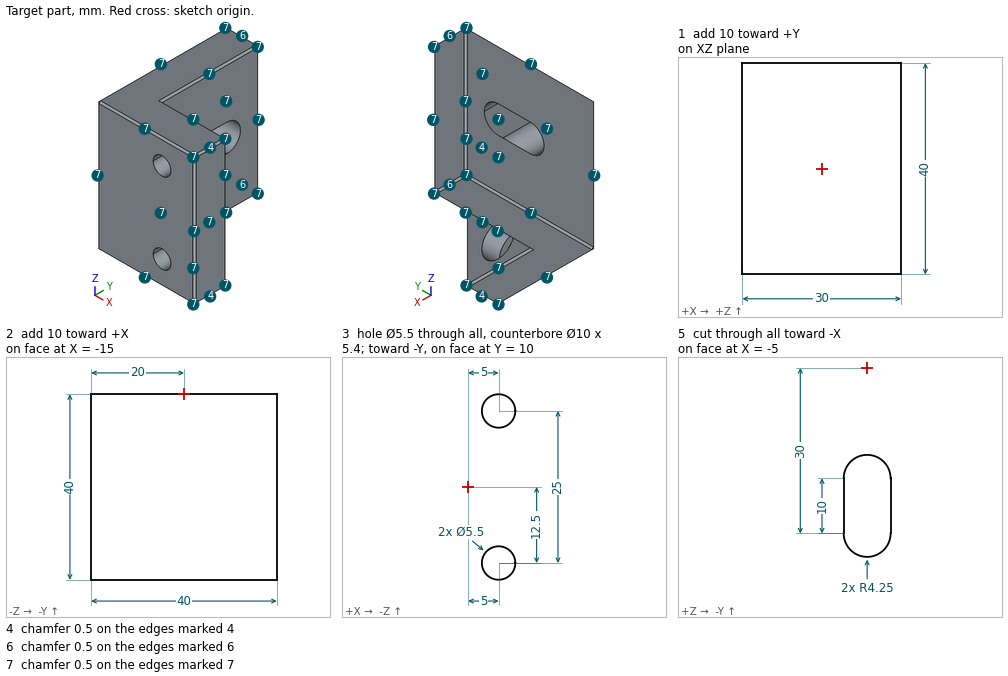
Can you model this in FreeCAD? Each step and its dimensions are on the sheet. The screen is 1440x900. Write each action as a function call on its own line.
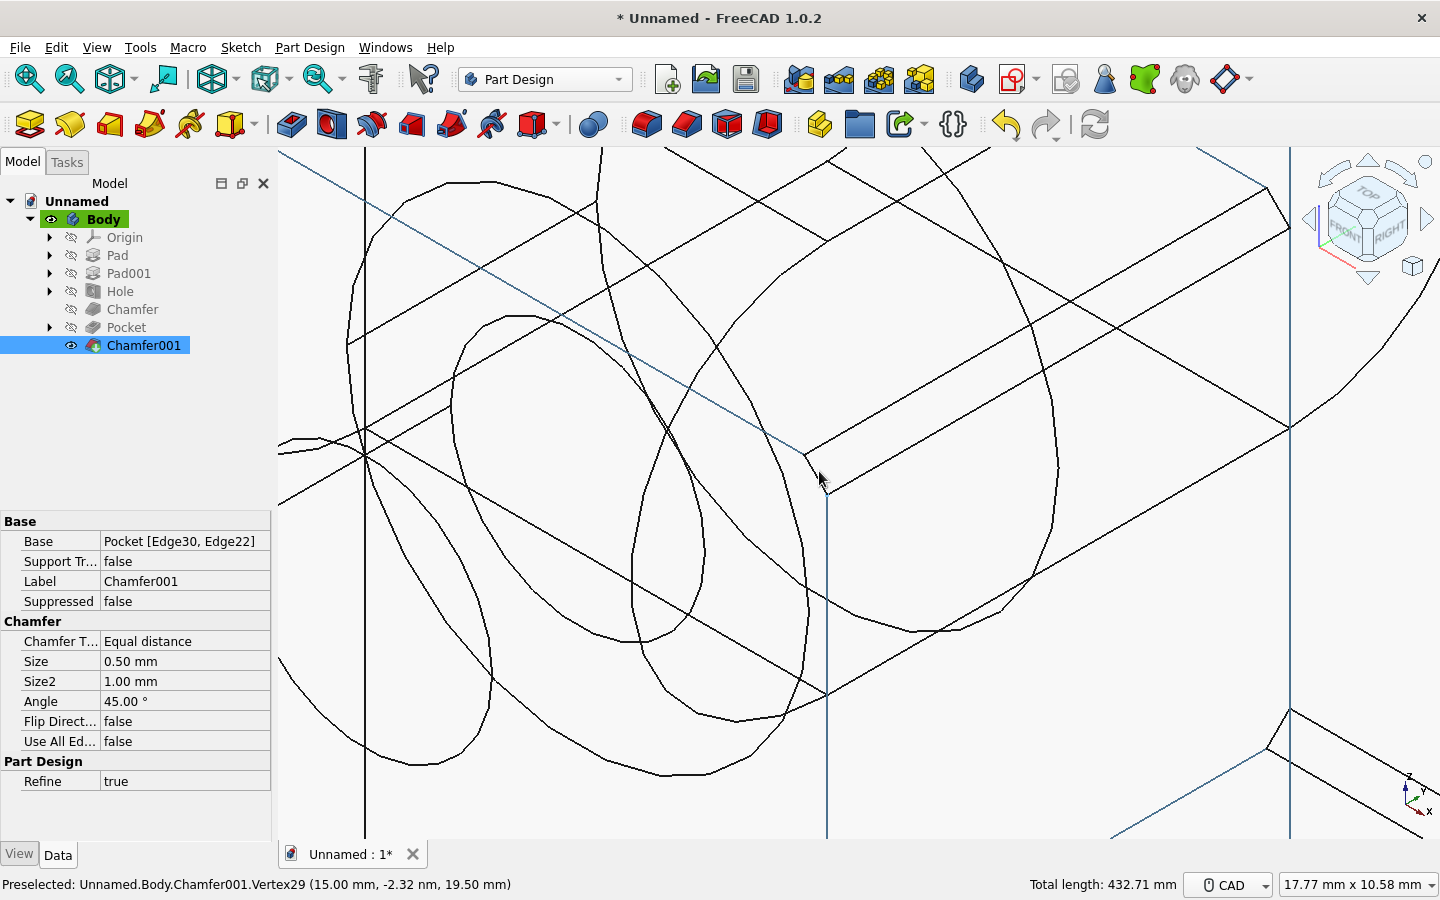
click(816, 474, ctrl)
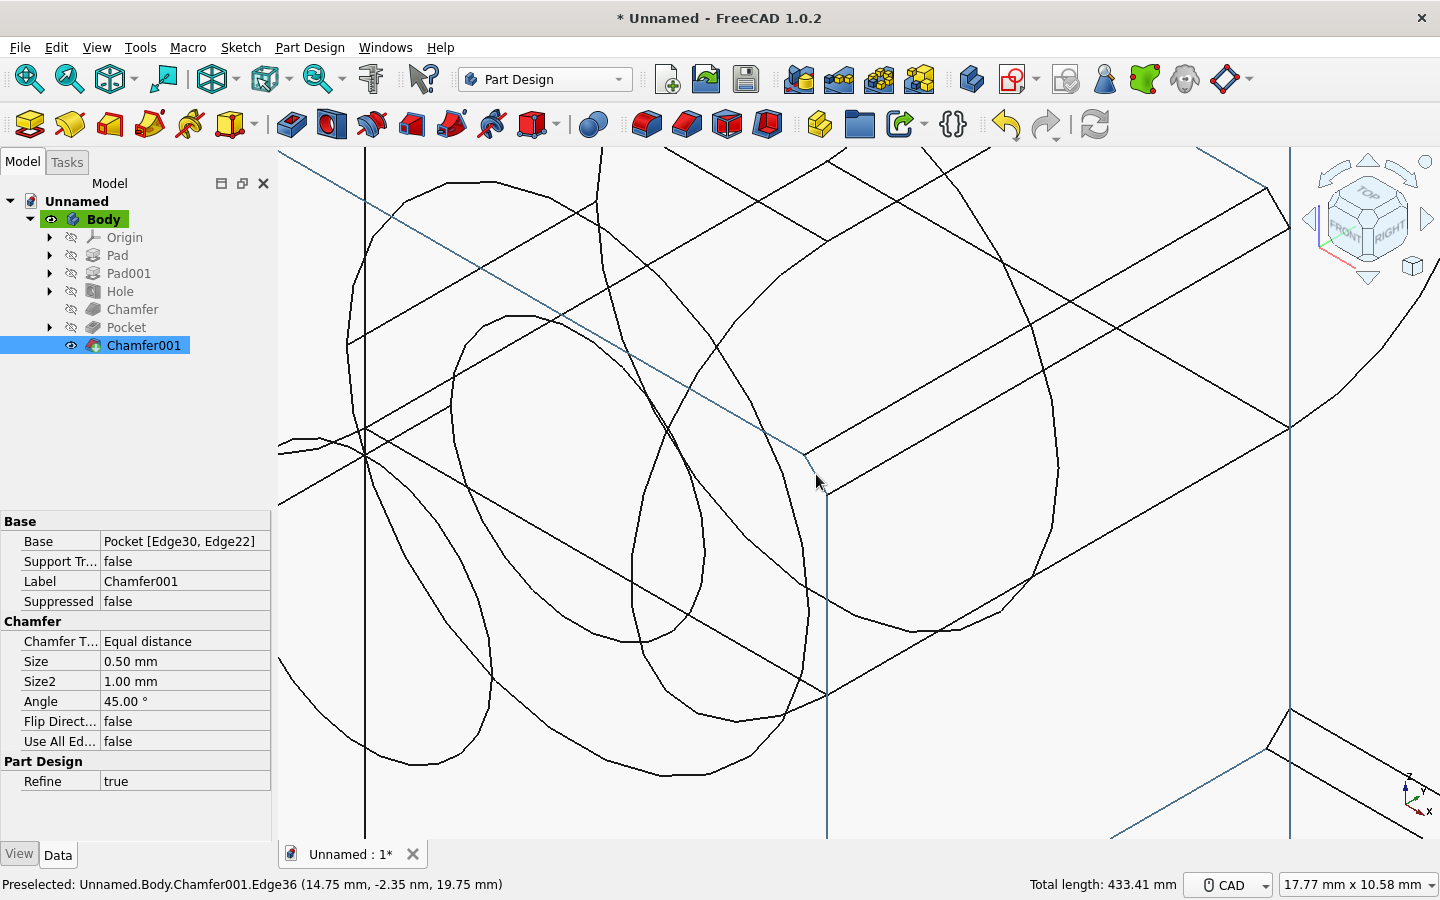
click(1274, 199, ctrl)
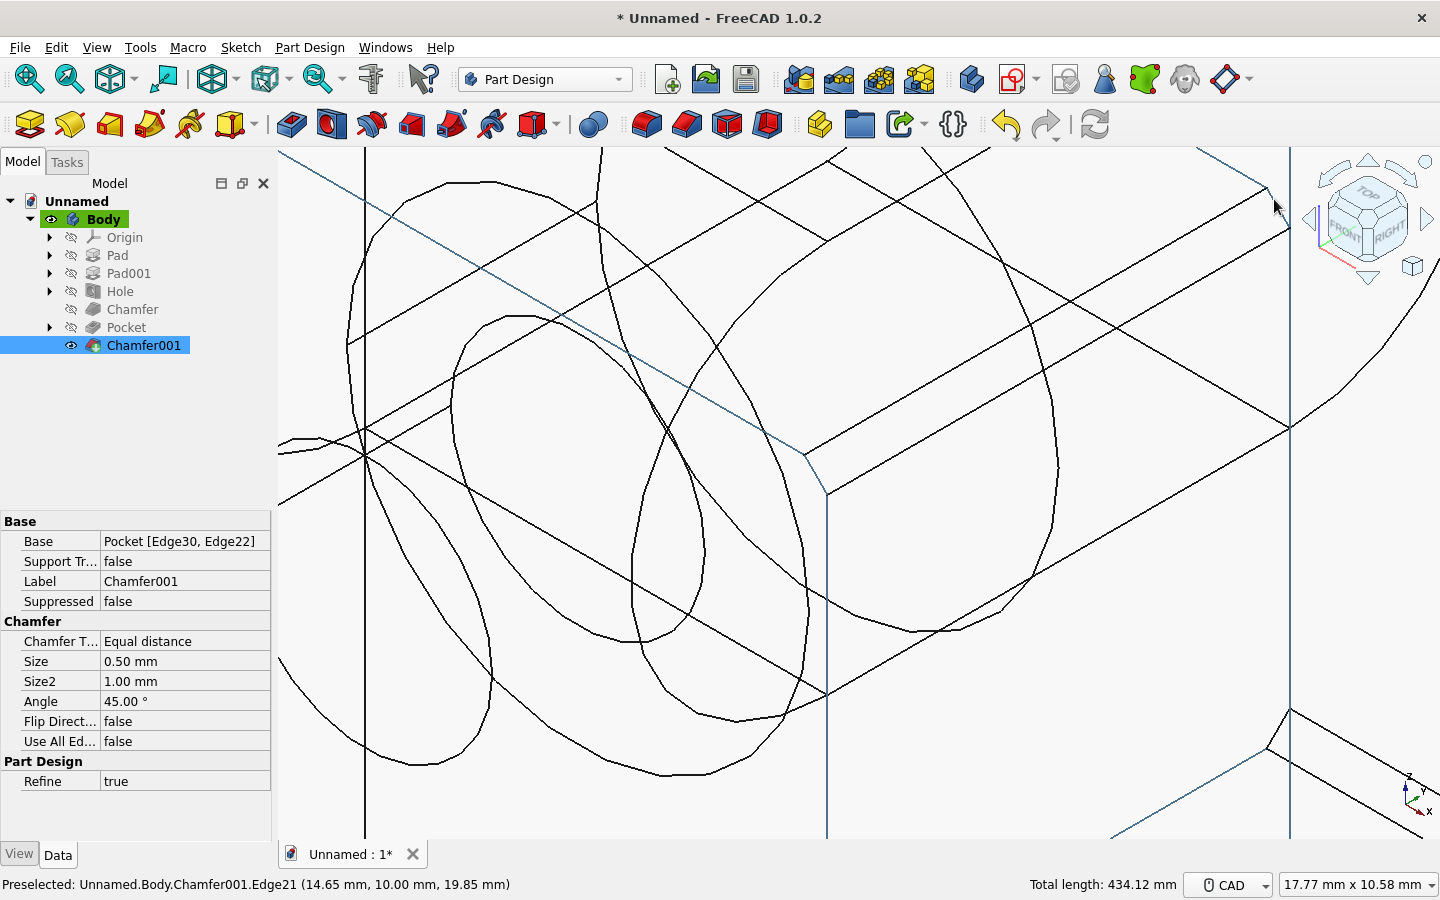
click(1278, 728, ctrl)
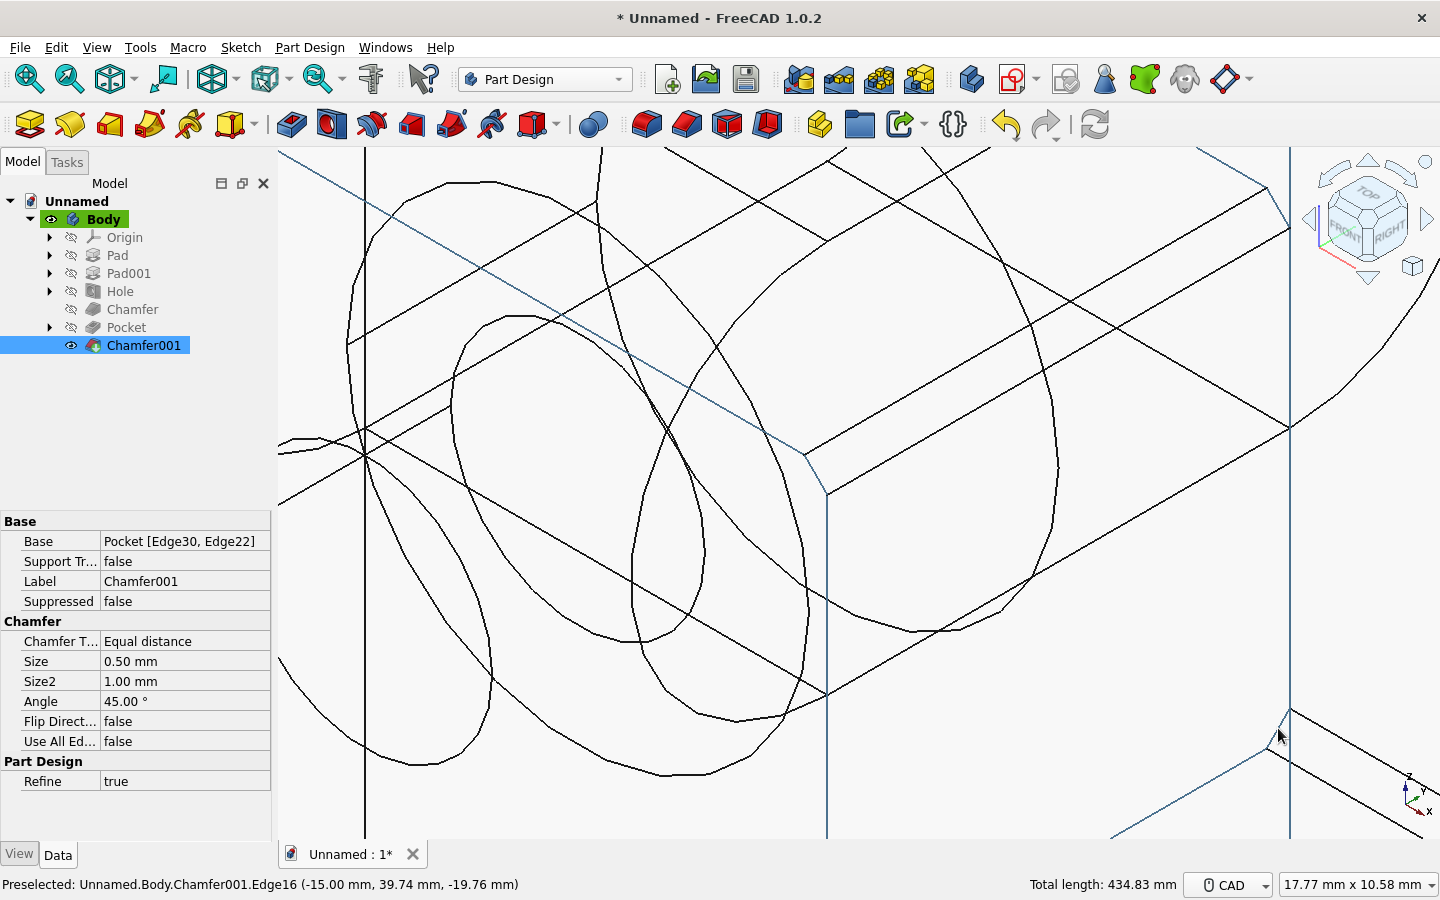
click(30, 80)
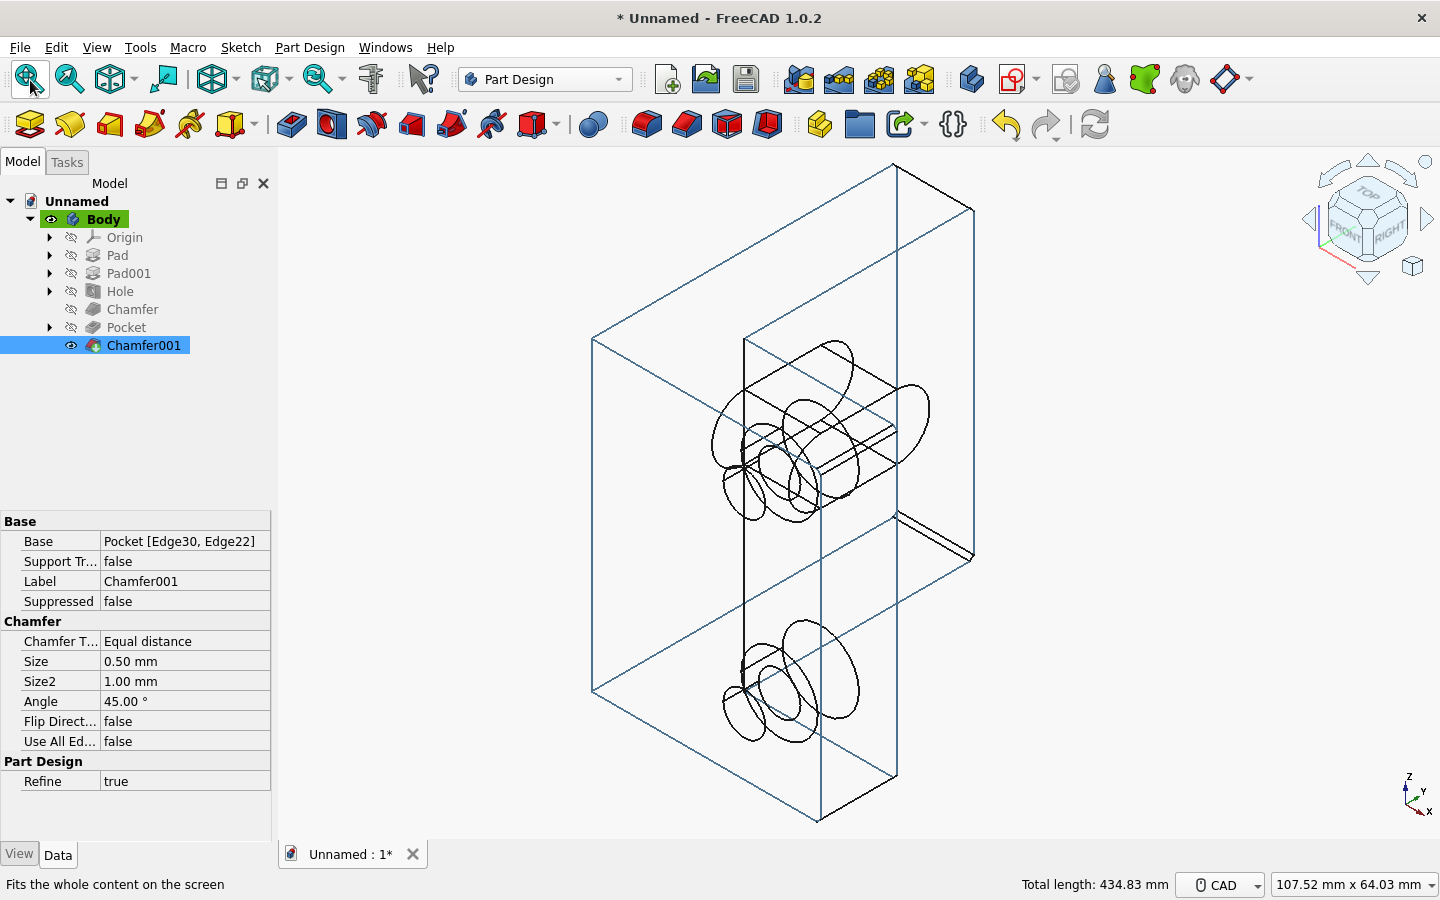
key(2)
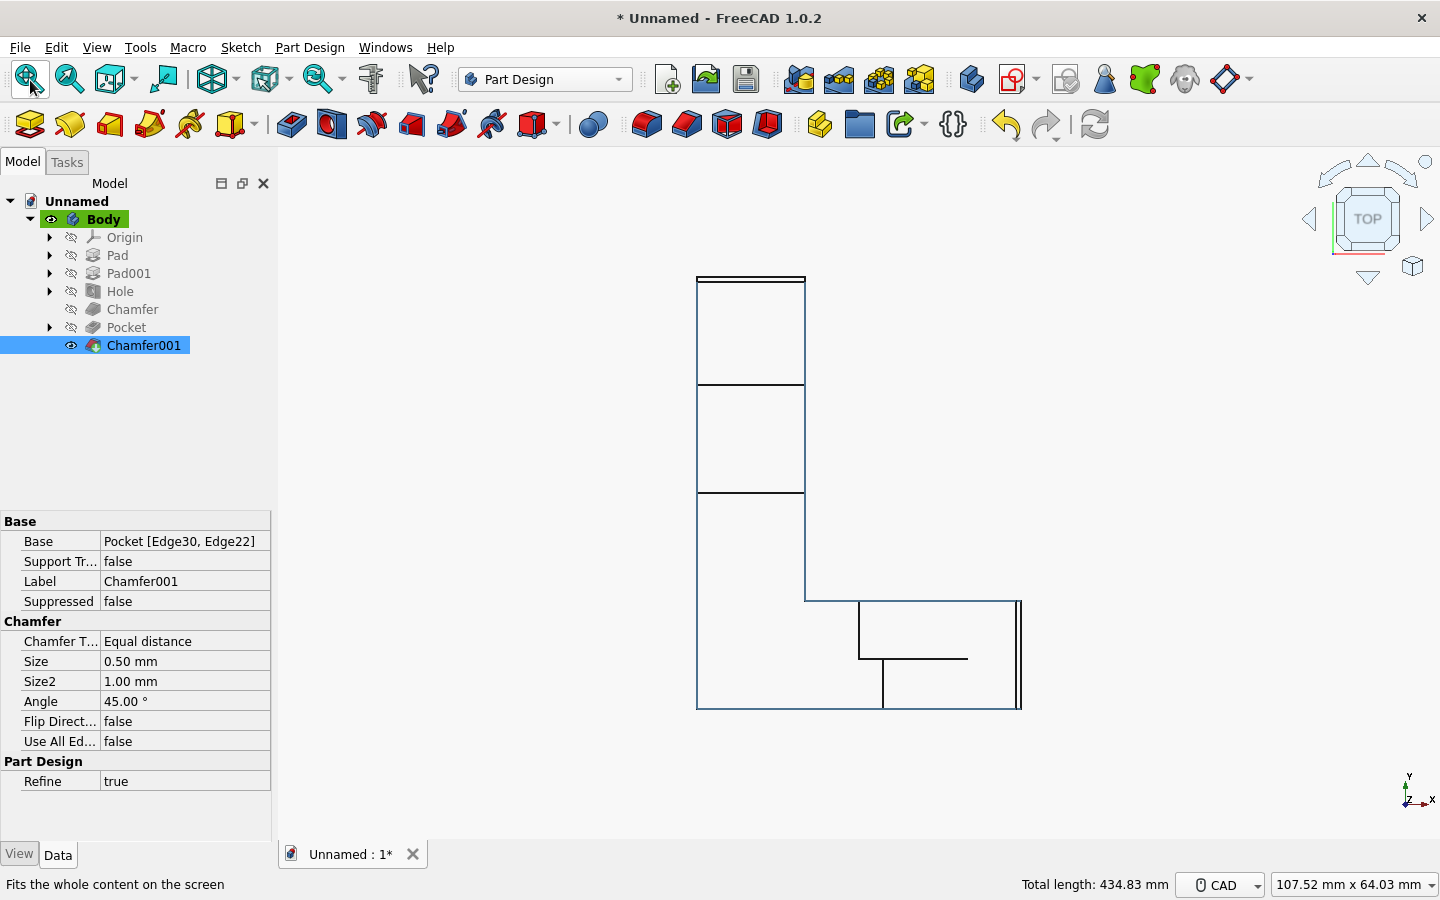
scroll(1018, 600, up, 9)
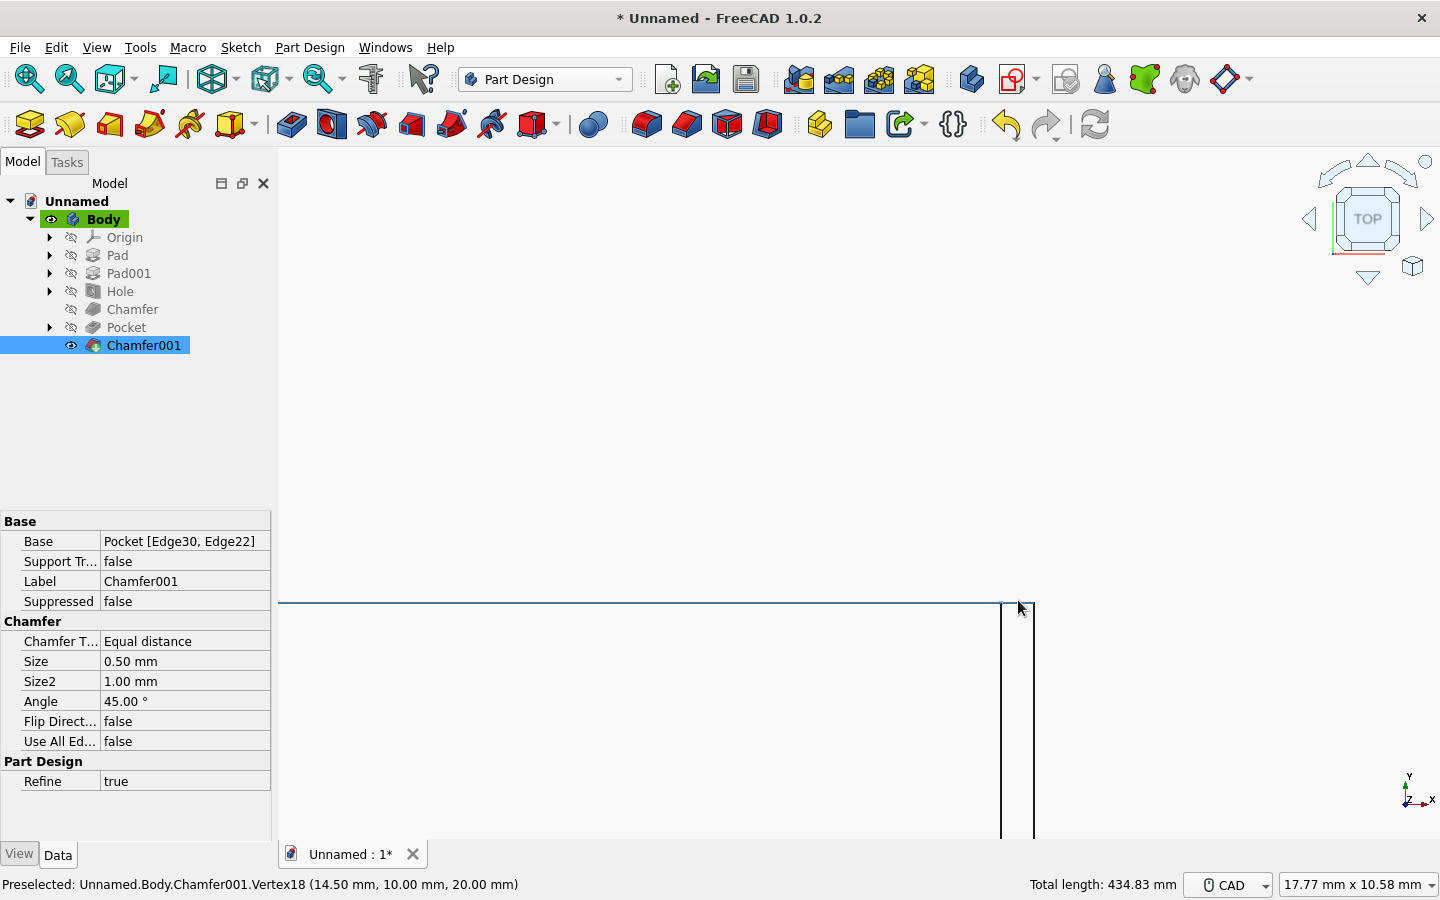
click(30, 80)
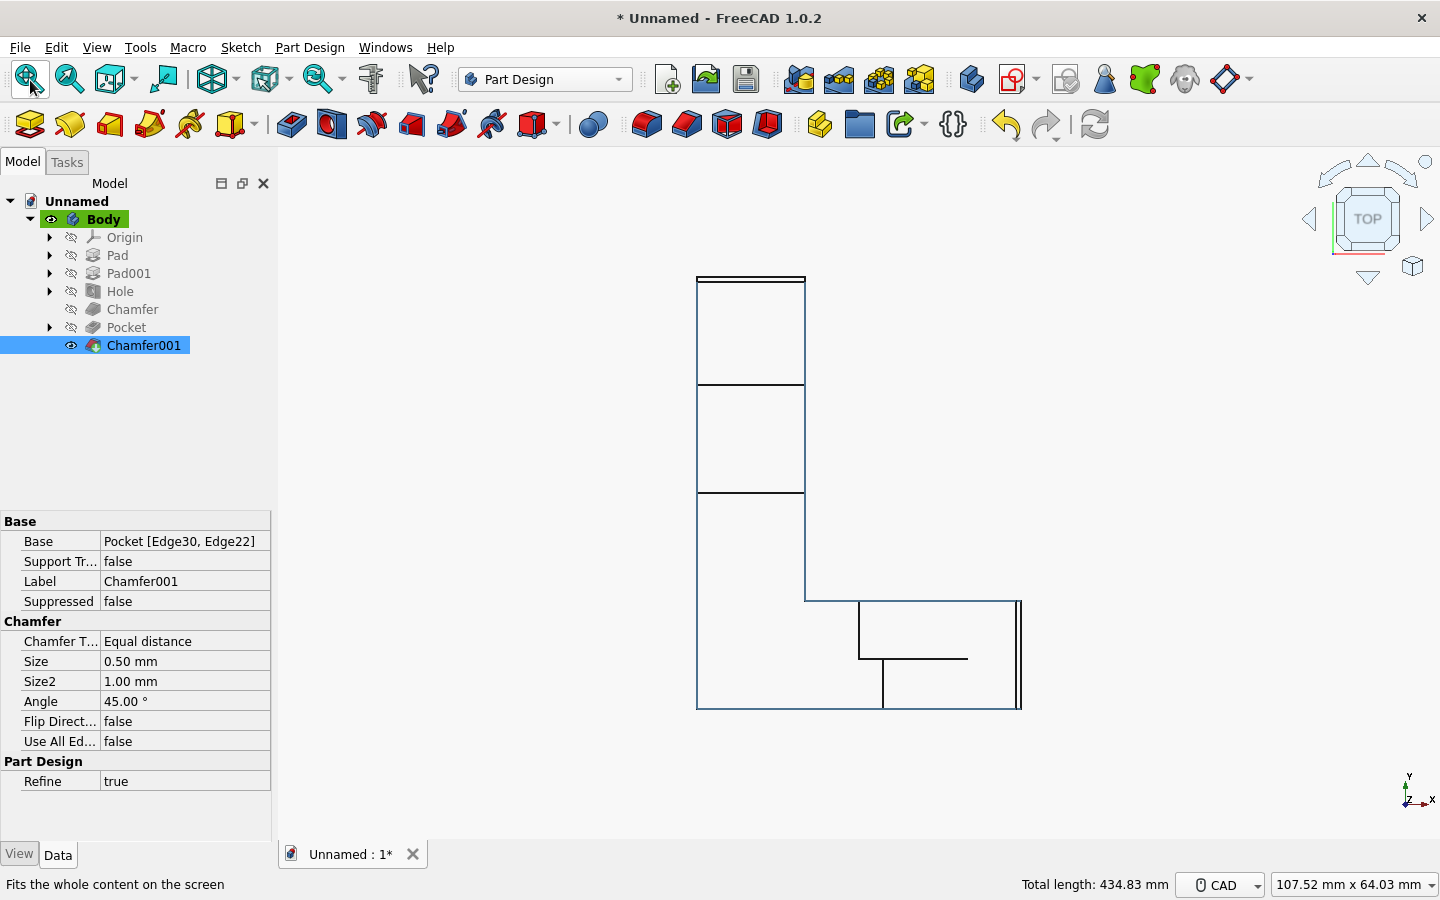
key(1)